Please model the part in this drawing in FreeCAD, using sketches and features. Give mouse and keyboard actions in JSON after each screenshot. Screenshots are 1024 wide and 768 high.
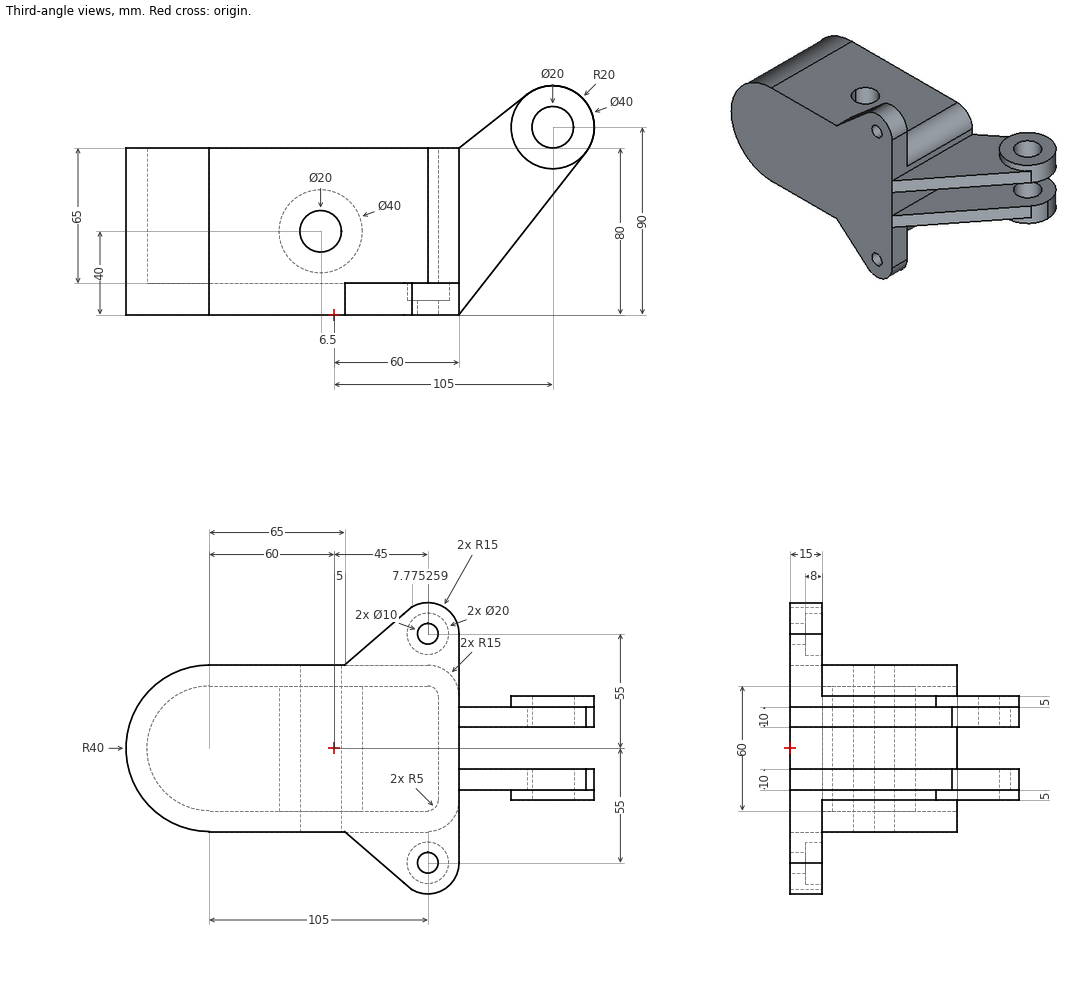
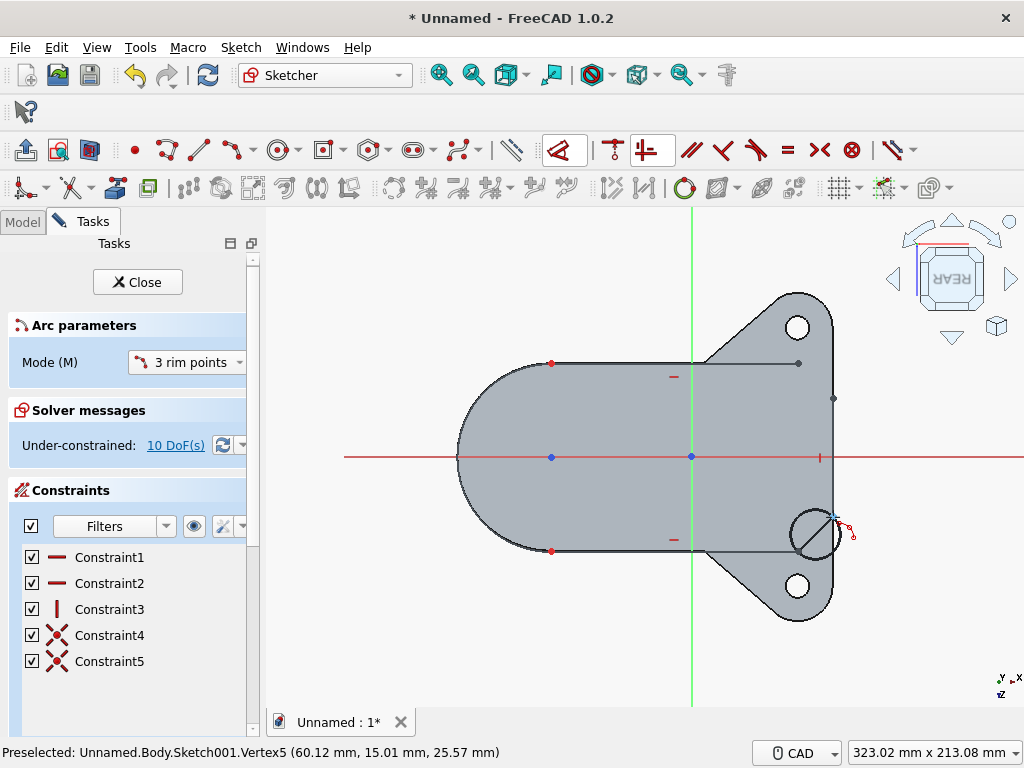
{"action": "scroll", "coordinate": [822, 541], "scroll_direction": "up", "scroll_amount": 3}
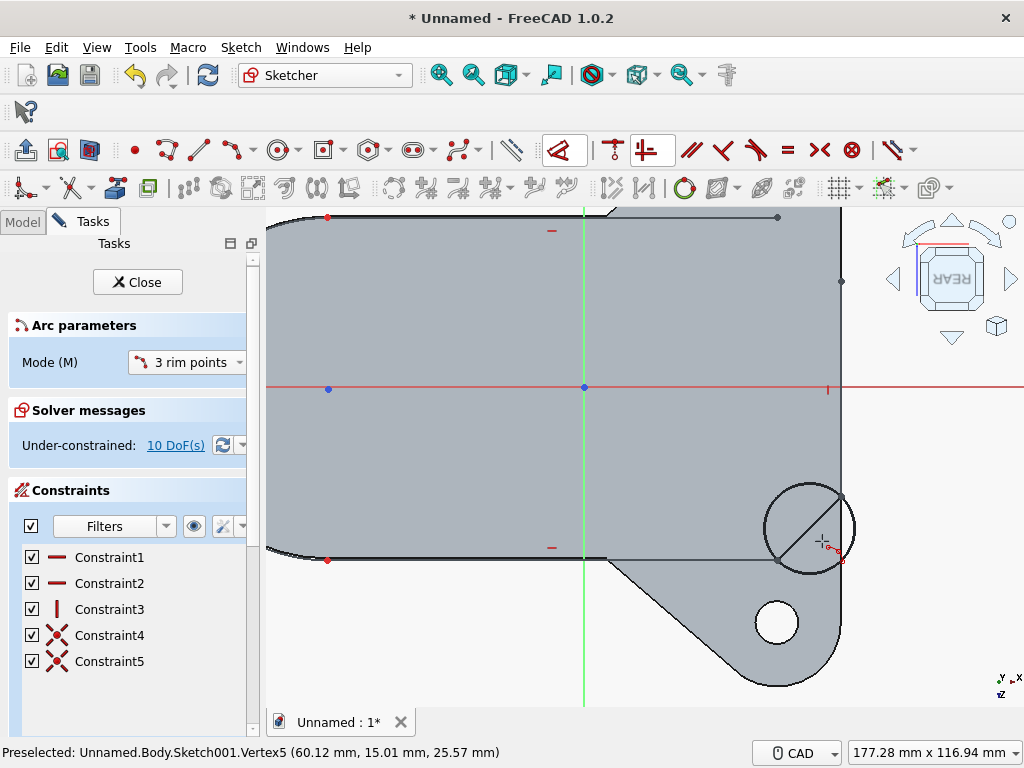
{"action": "left_click", "coordinate": [822, 540]}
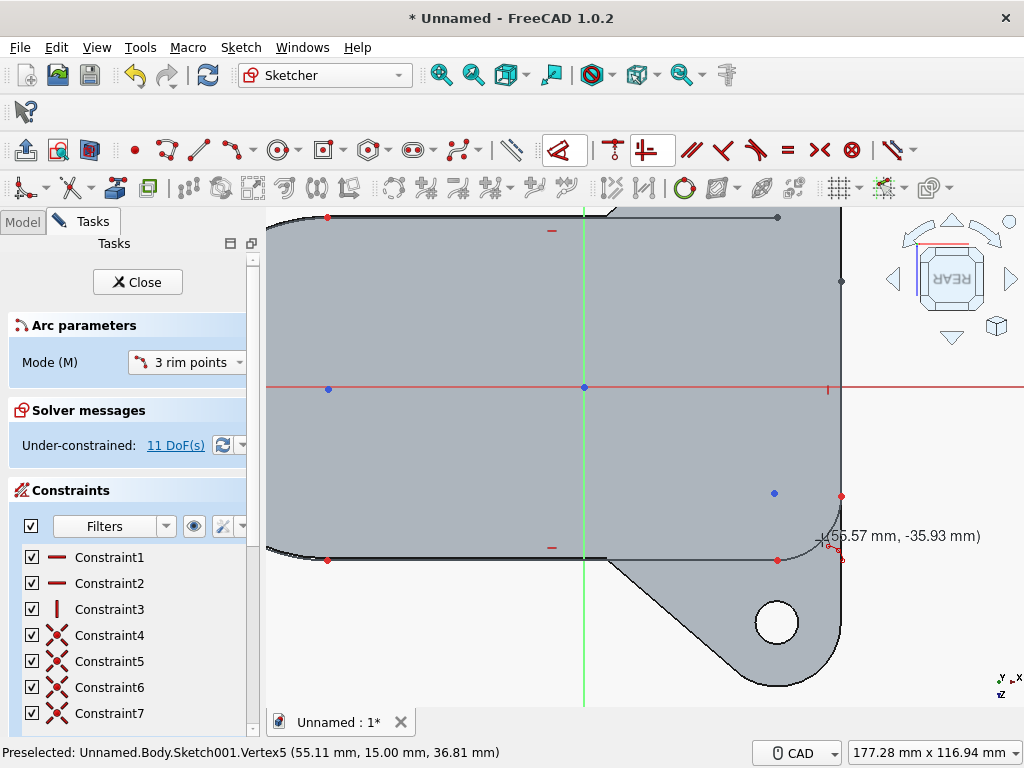
{"action": "left_click", "coordinate": [841, 282]}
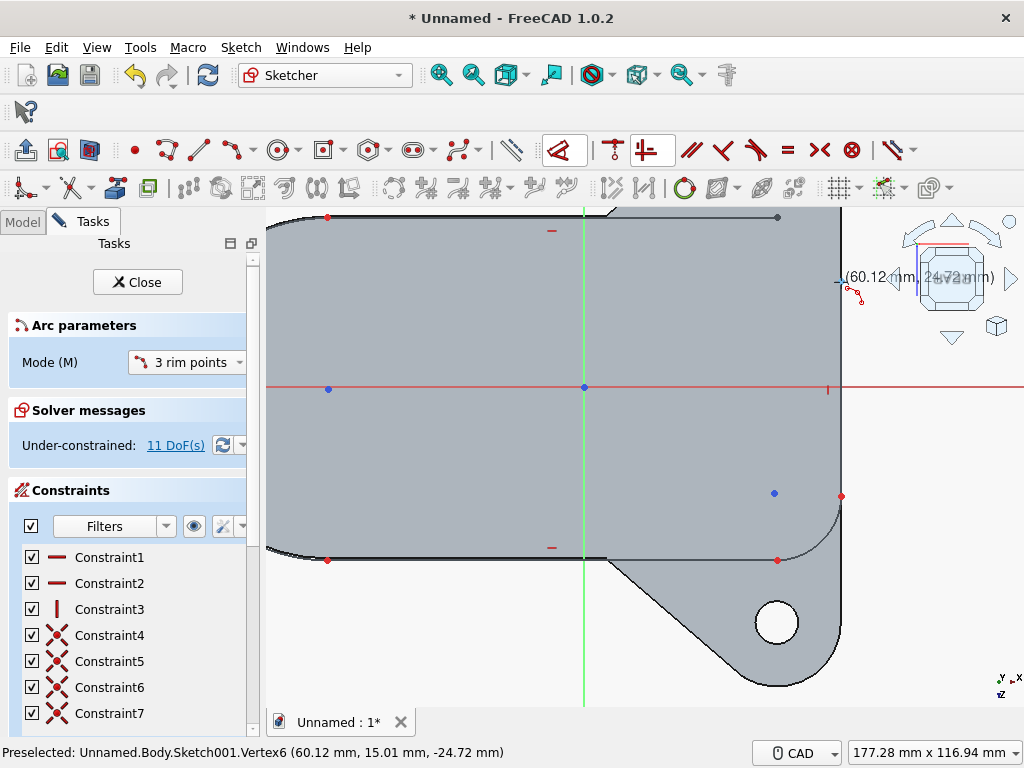
{"action": "scroll", "coordinate": [671, 542], "scroll_direction": "down", "scroll_amount": 3}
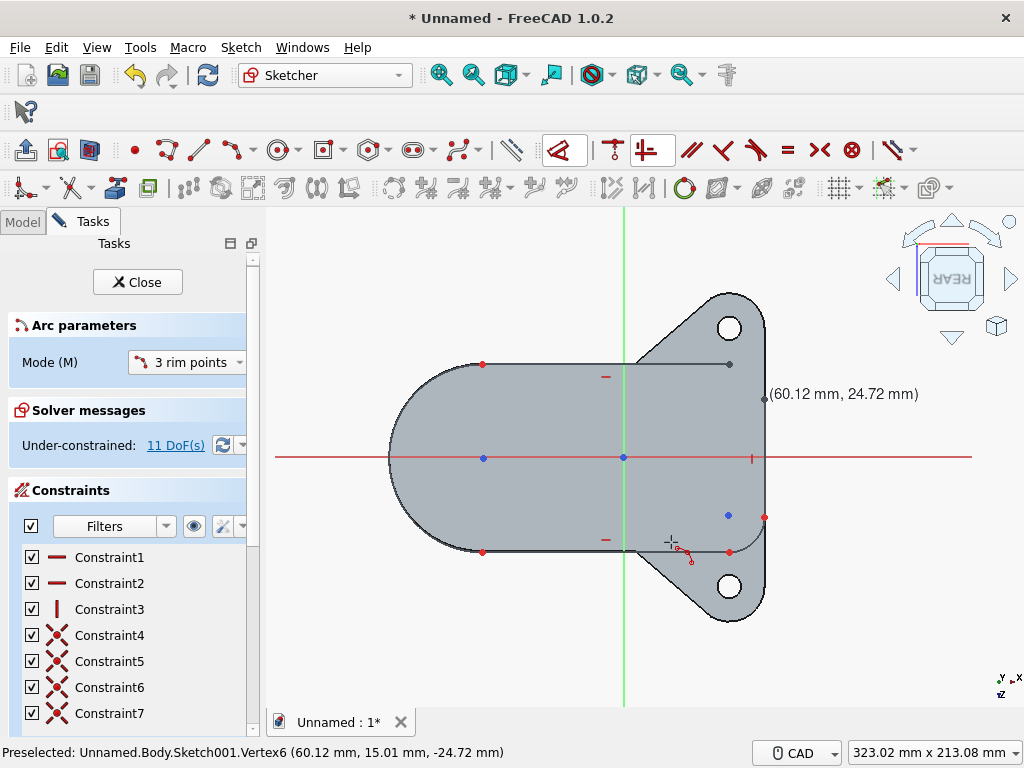
{"action": "left_click", "coordinate": [730, 364]}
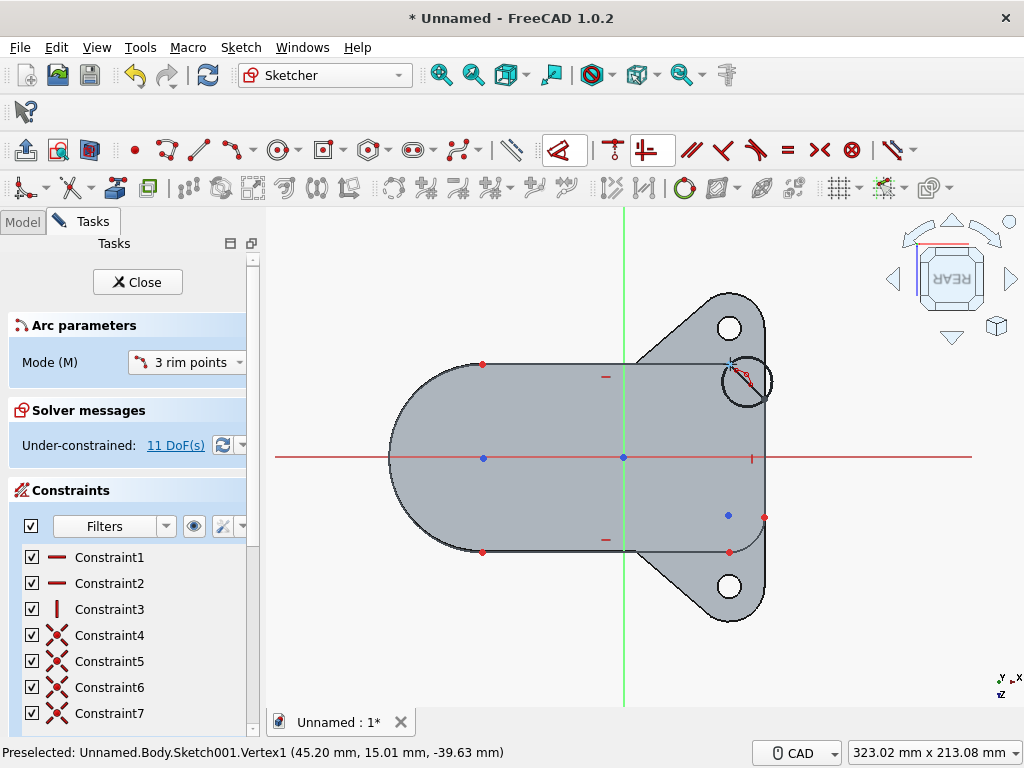
{"action": "scroll", "coordinate": [754, 374], "scroll_direction": "up", "scroll_amount": 3}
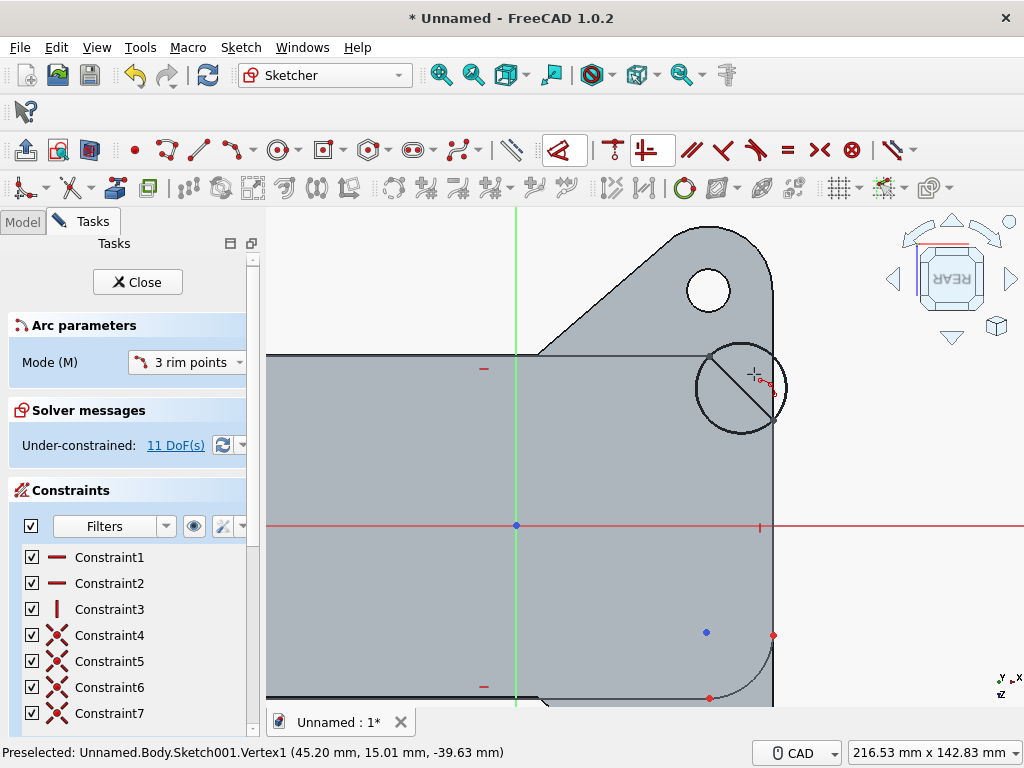
{"action": "left_click", "coordinate": [754, 374]}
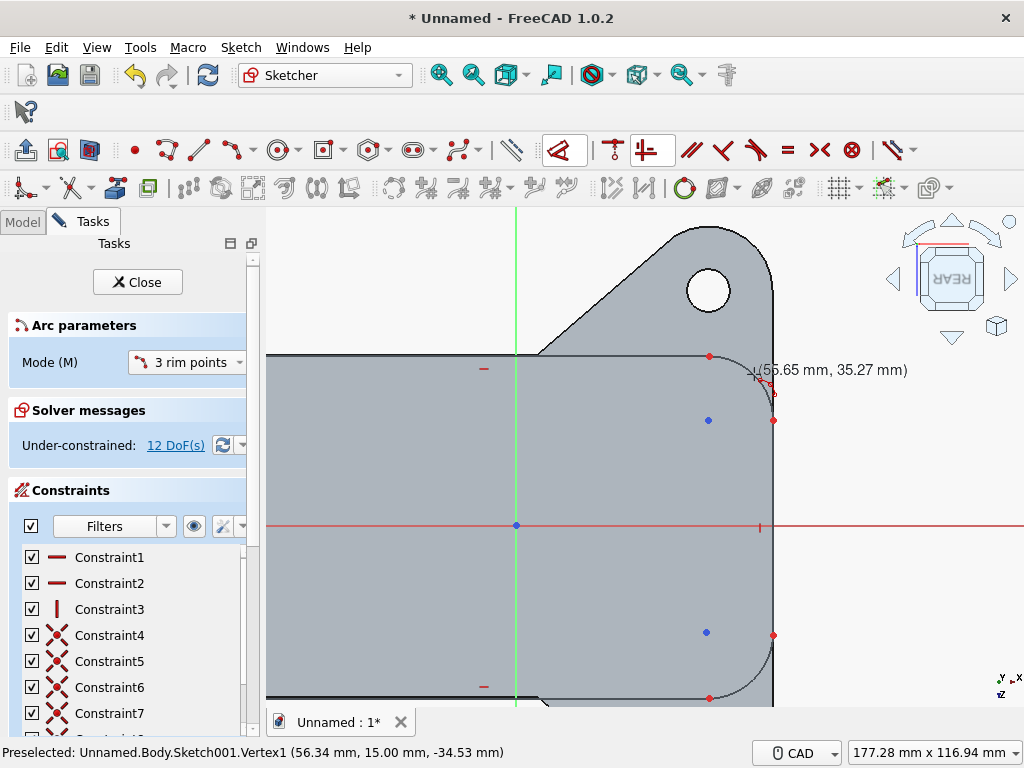
{"action": "left_click", "coordinate": [200, 150]}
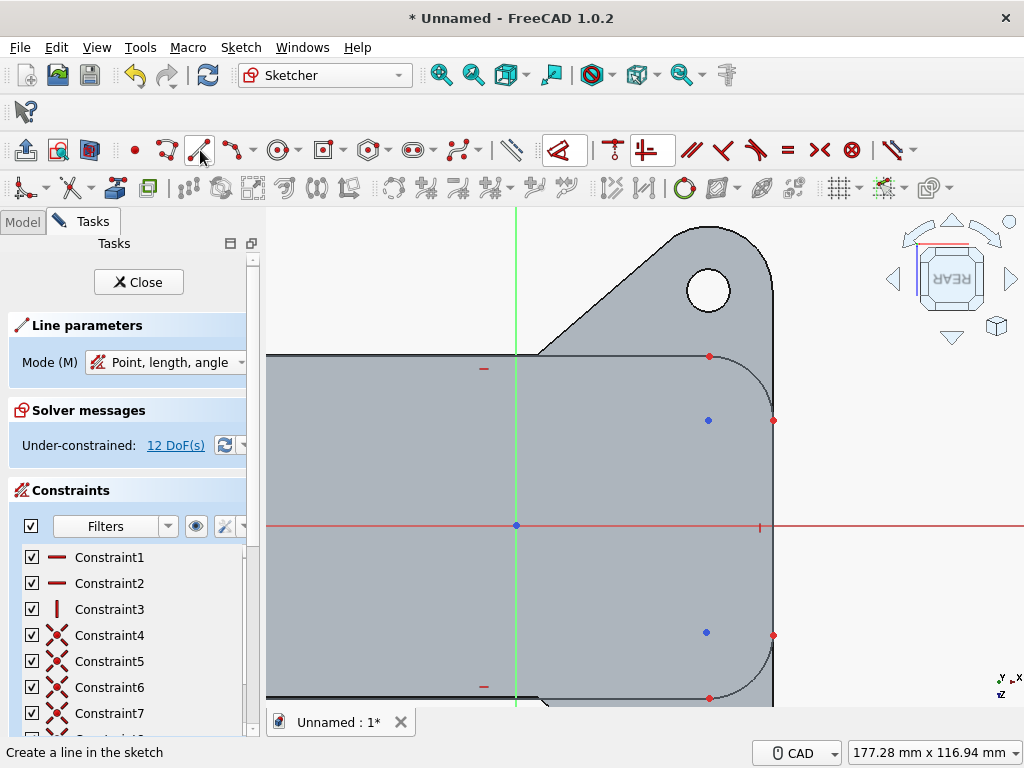
{"action": "scroll", "coordinate": [754, 373], "scroll_direction": "down", "scroll_amount": 3}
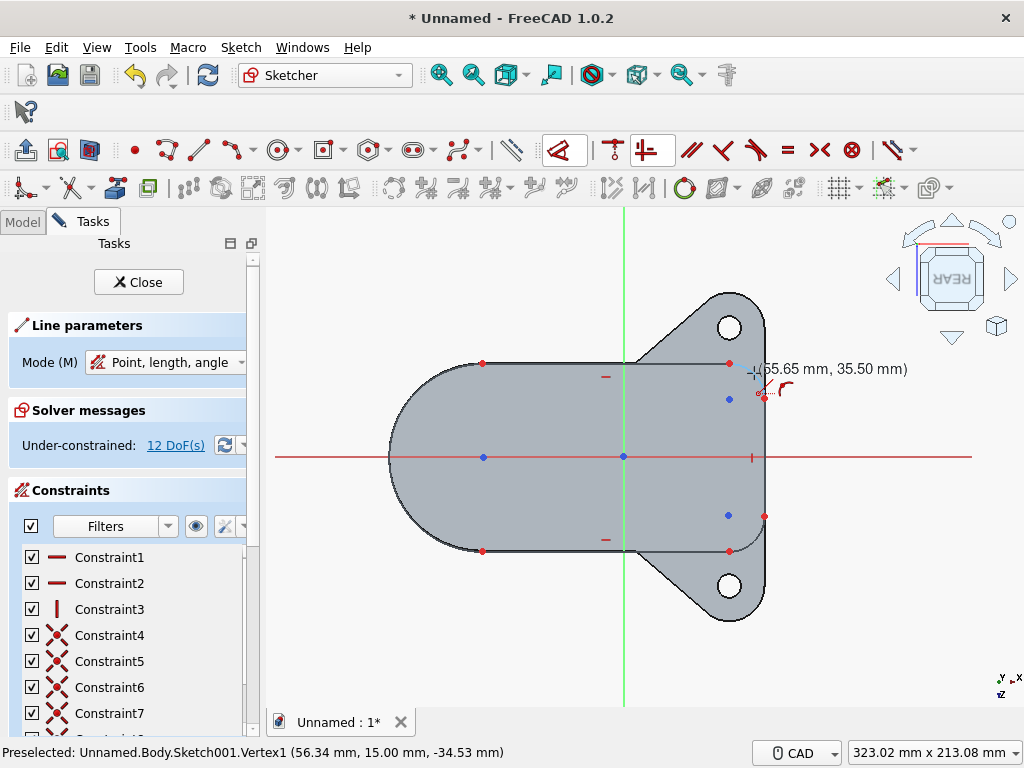
{"action": "left_click", "coordinate": [483, 387]}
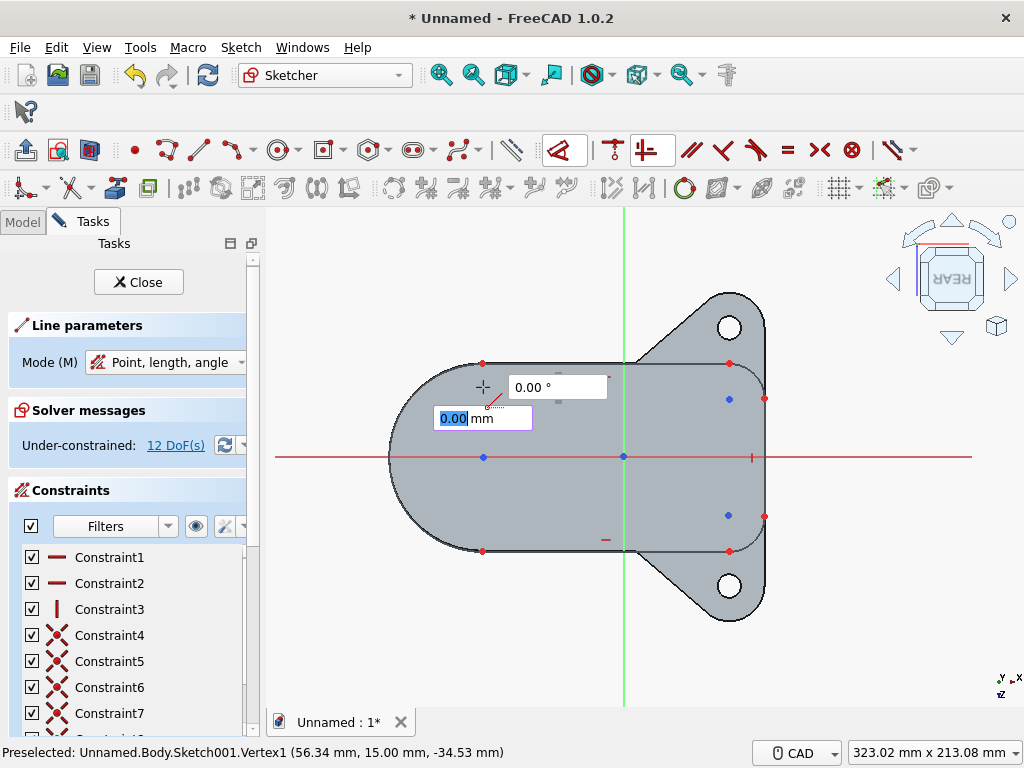
{"action": "scroll", "coordinate": [729, 387], "scroll_direction": "up", "scroll_amount": 2}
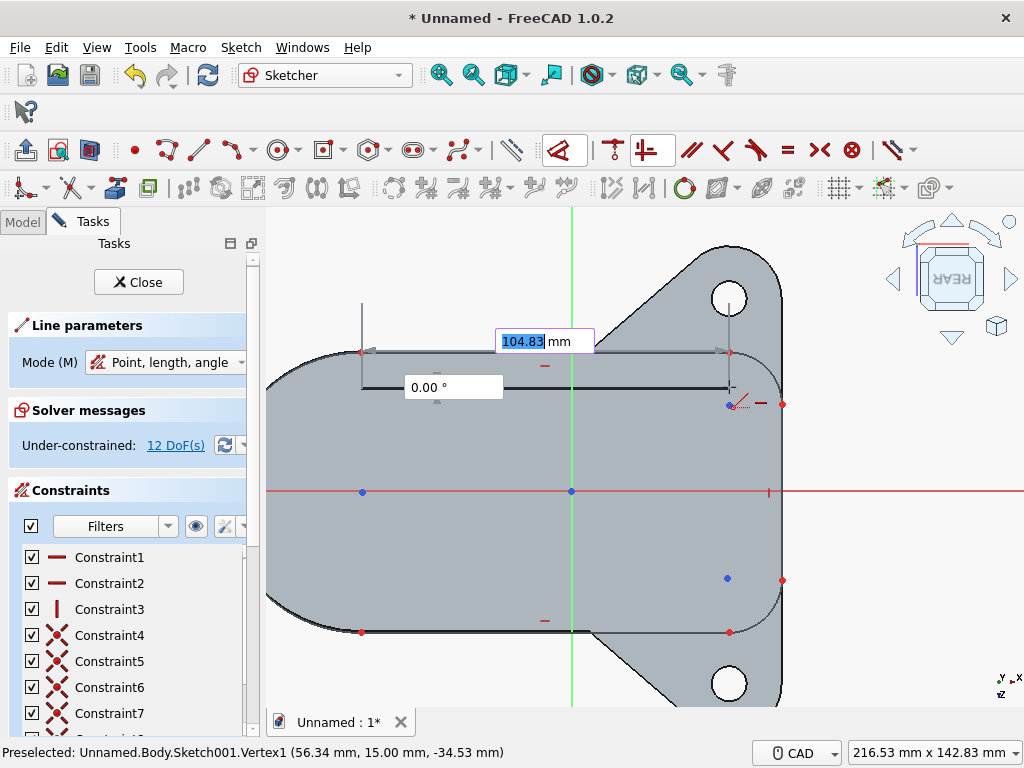
{"action": "left_click", "coordinate": [729, 387]}